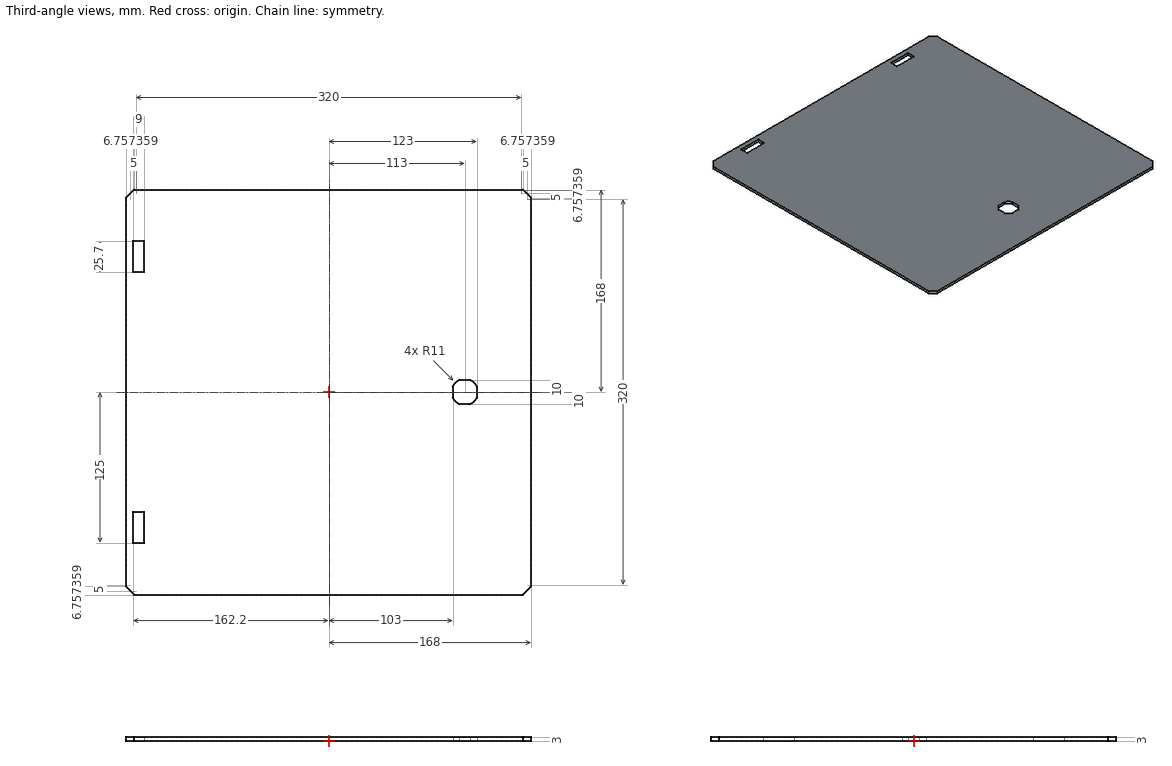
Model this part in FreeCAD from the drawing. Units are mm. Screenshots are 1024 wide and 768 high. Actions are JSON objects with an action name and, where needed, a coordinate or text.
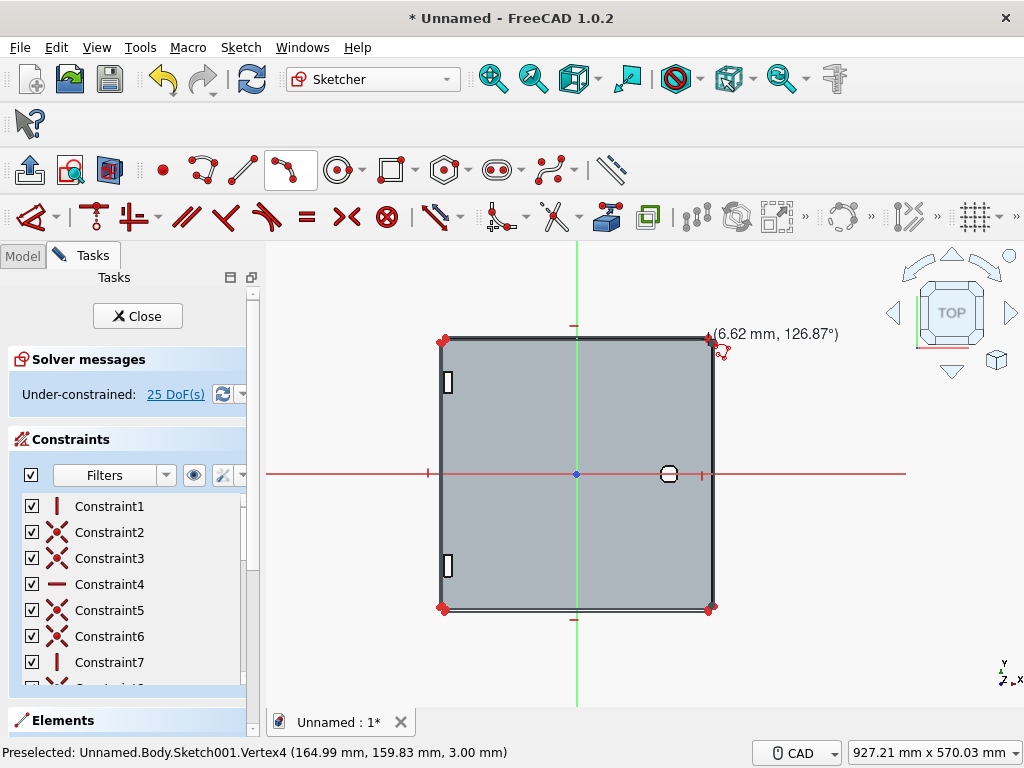
{"action": "scroll", "coordinate": [712, 605], "scroll_direction": "up", "scroll_amount": 10}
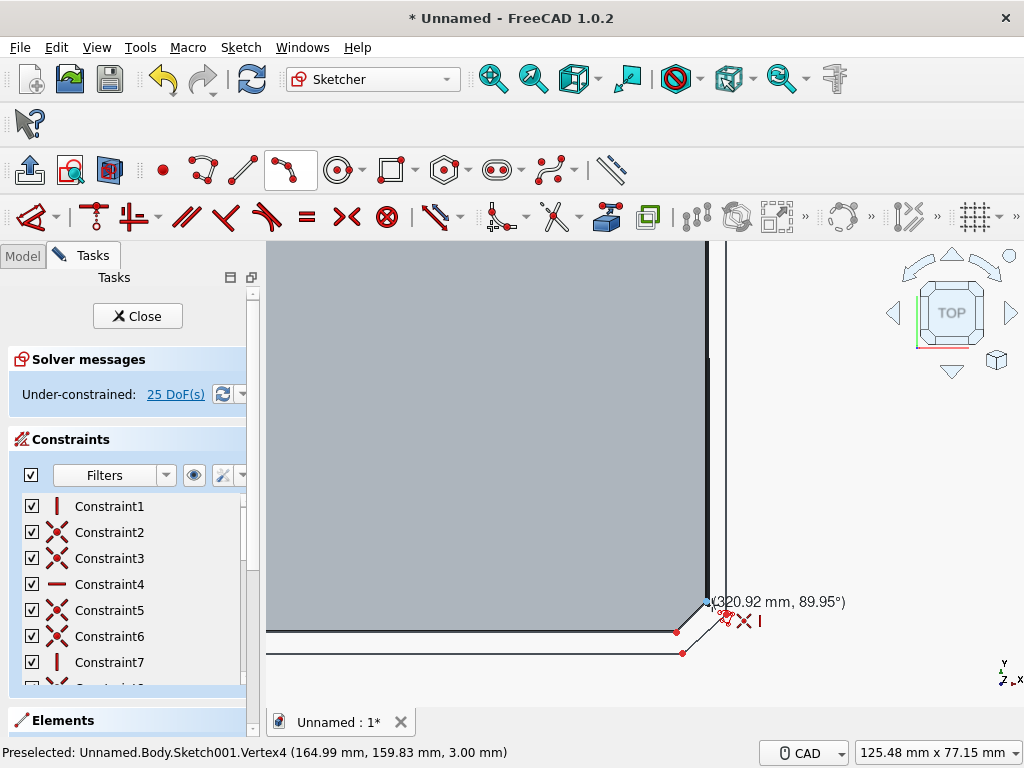
{"action": "left_click", "coordinate": [707, 601]}
{"action": "key", "text": "Escape"}
{"action": "key", "text": "Escape"}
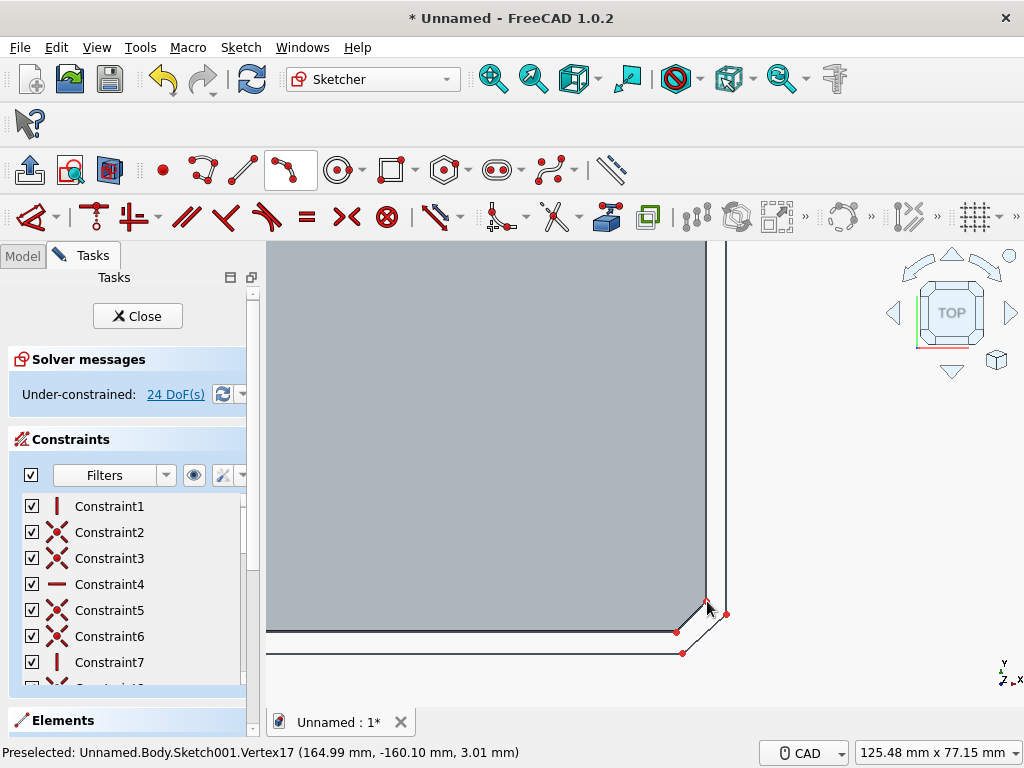
{"action": "scroll", "coordinate": [712, 605], "scroll_direction": "down", "scroll_amount": 10}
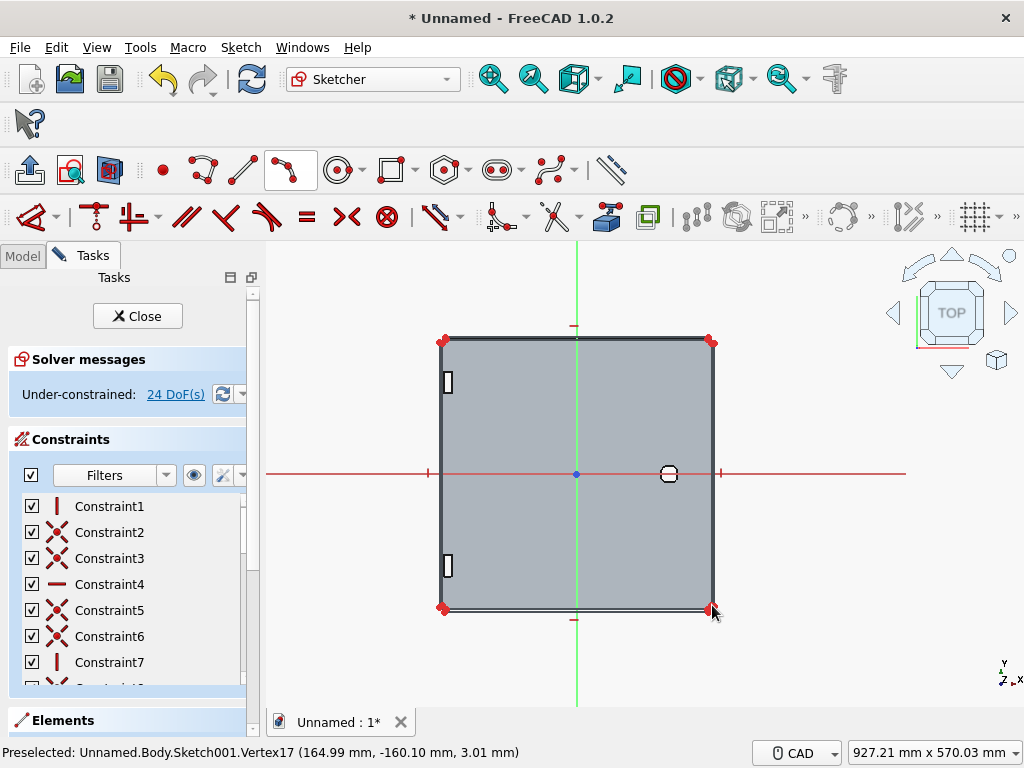
{"action": "scroll", "coordinate": [714, 343], "scroll_direction": "up", "scroll_amount": 8}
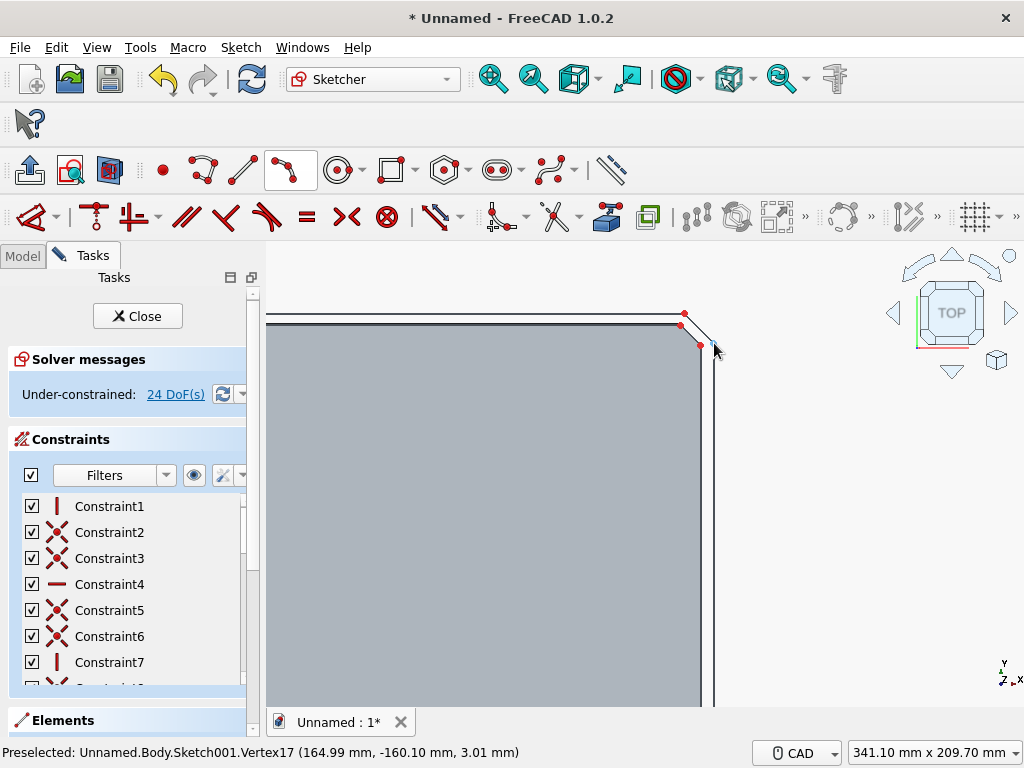
{"action": "left_click", "coordinate": [714, 344]}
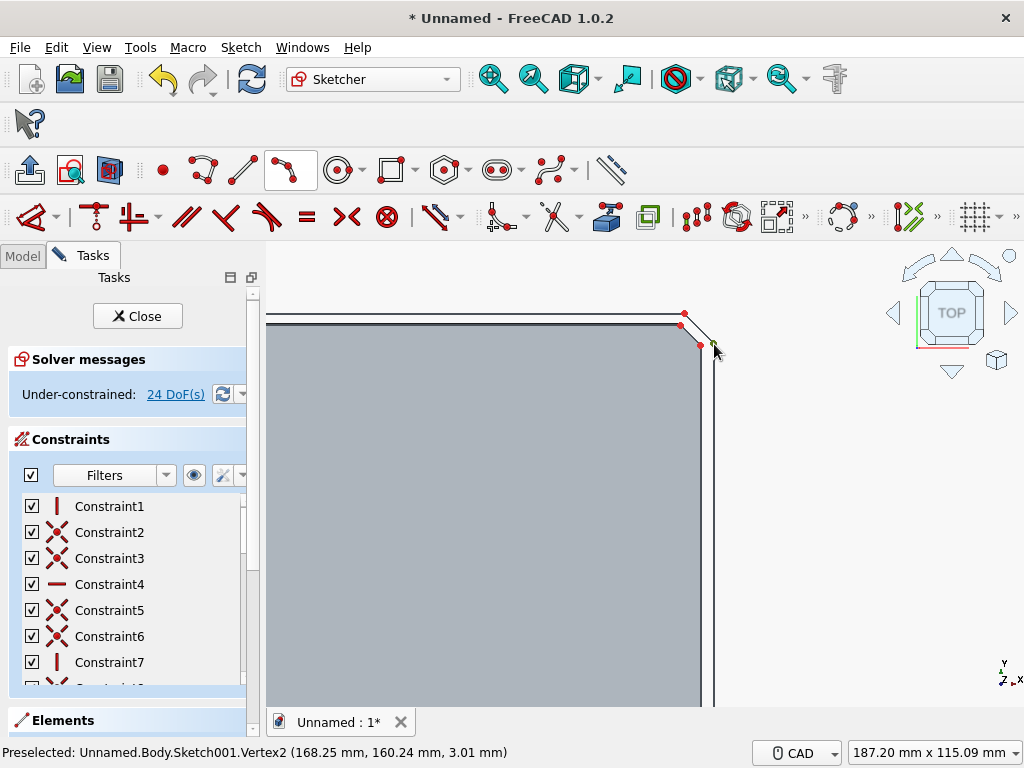
{"action": "scroll", "coordinate": [714, 343], "scroll_direction": "down", "scroll_amount": 8}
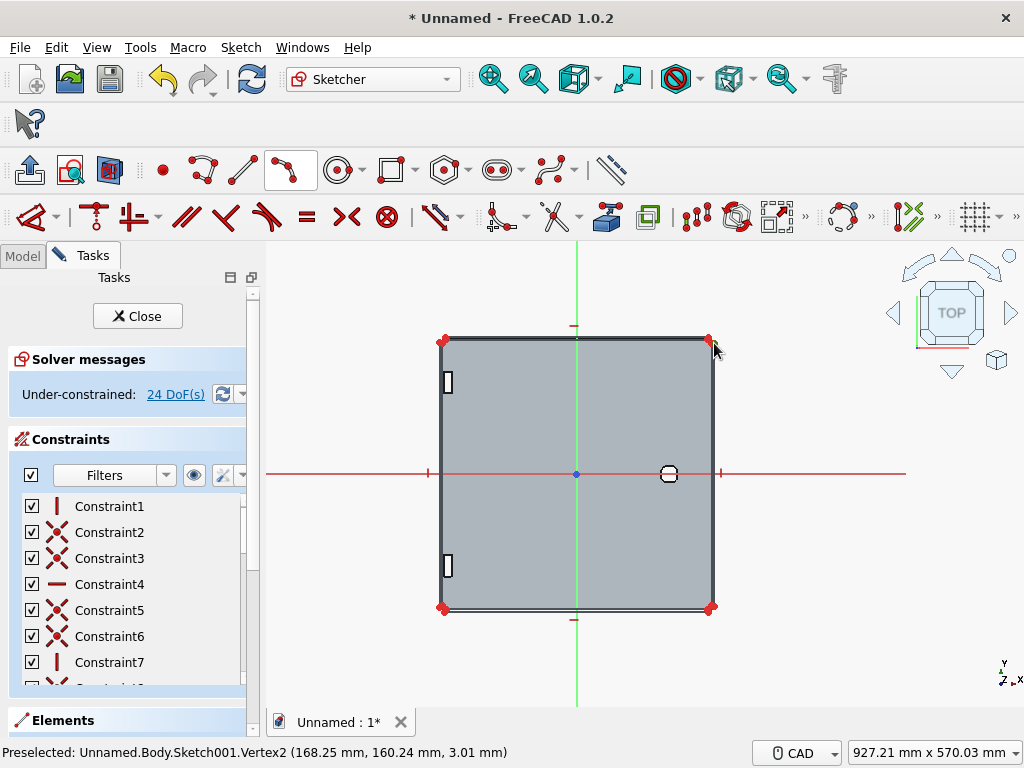
{"action": "scroll", "coordinate": [440, 343], "scroll_direction": "up", "scroll_amount": 9}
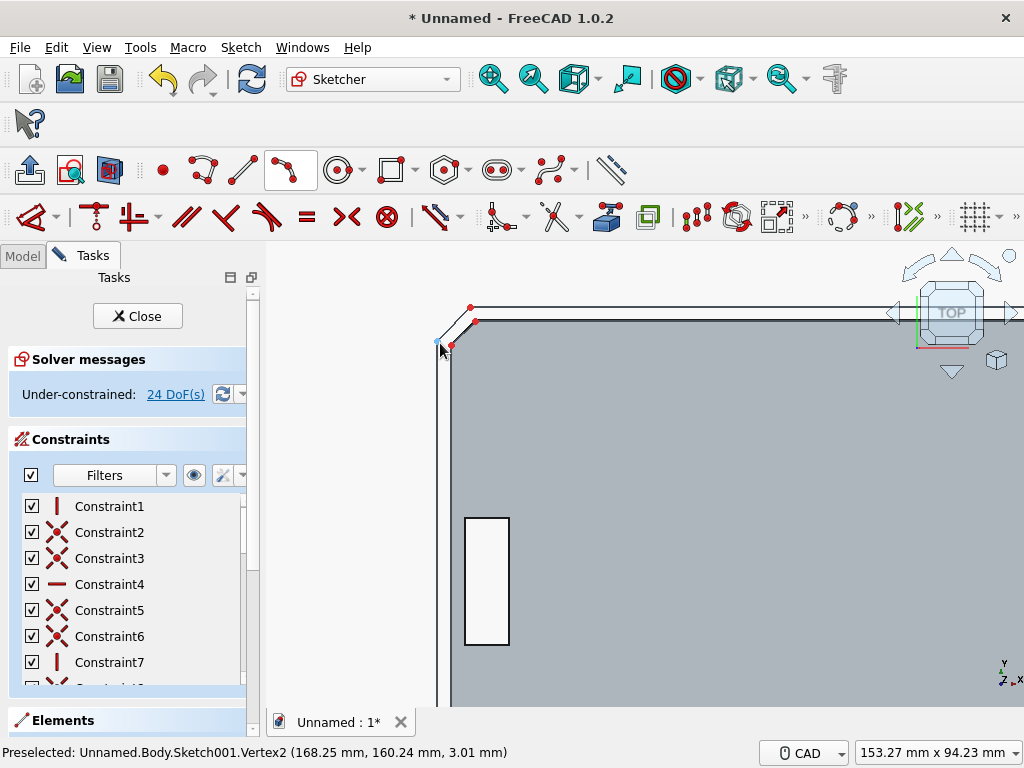
{"action": "left_click", "coordinate": [437, 342]}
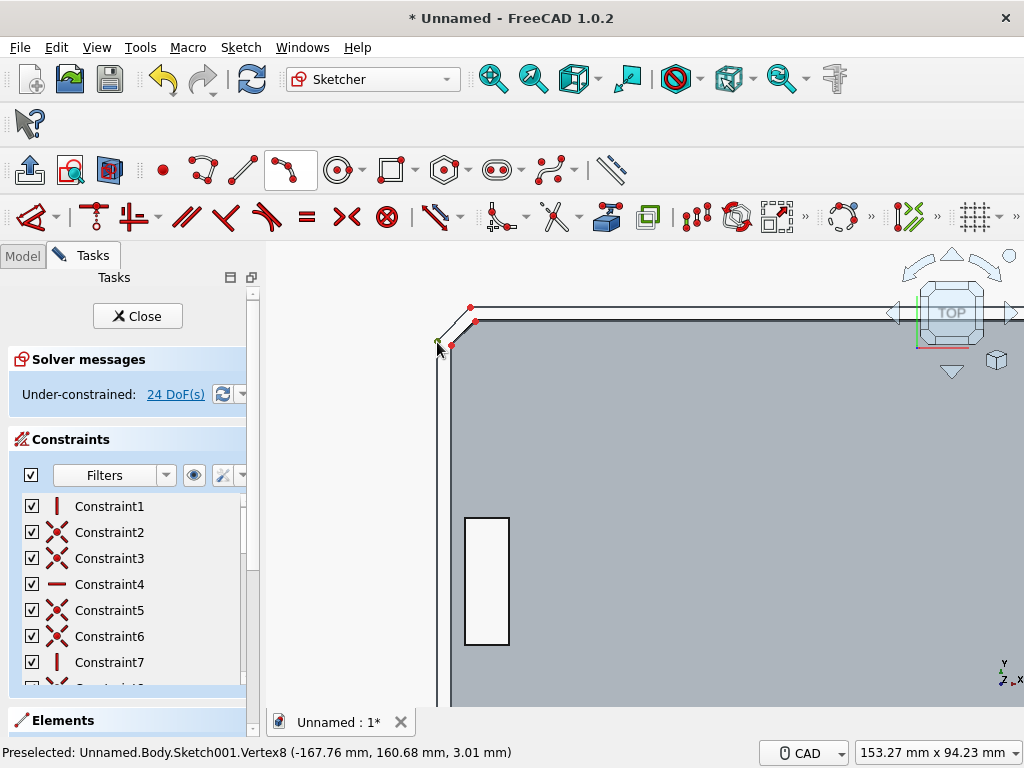
{"action": "scroll", "coordinate": [440, 343], "scroll_direction": "down", "scroll_amount": 9}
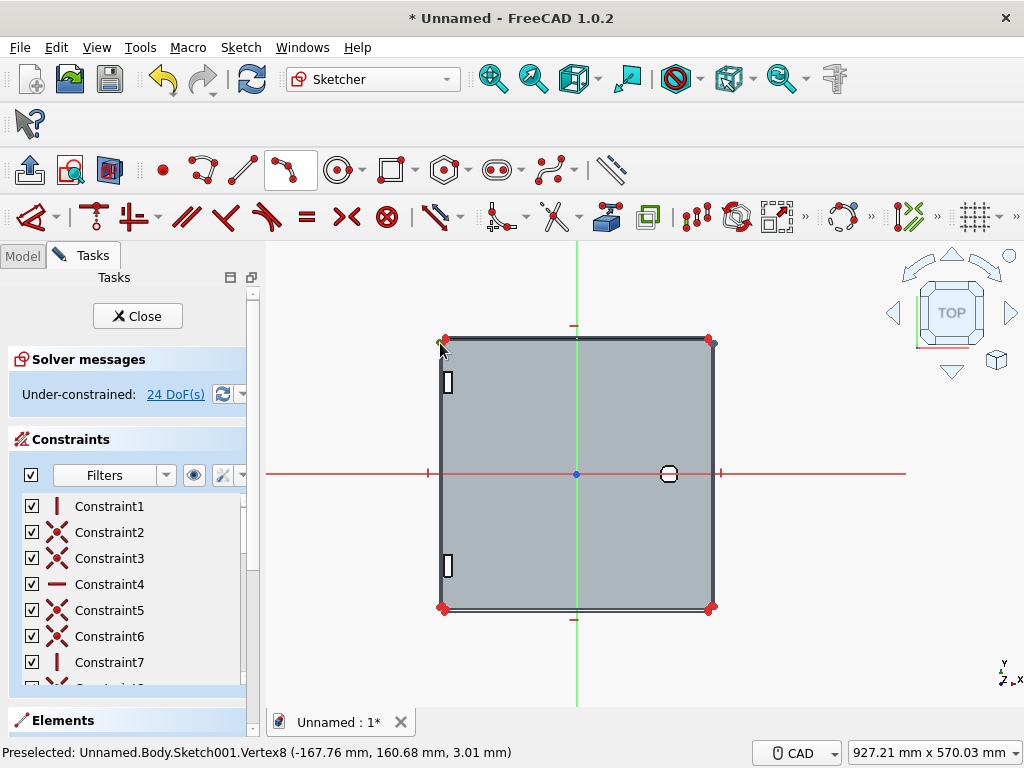
{"action": "left_click", "coordinate": [577, 650]}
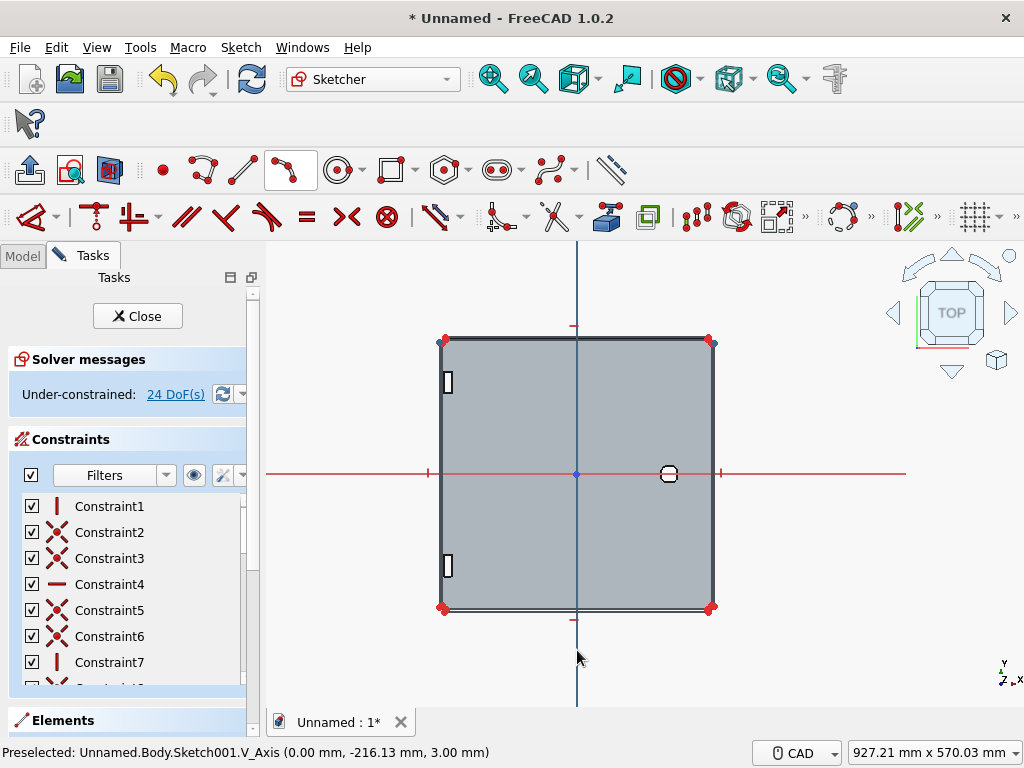
{"action": "left_click", "coordinate": [348, 218]}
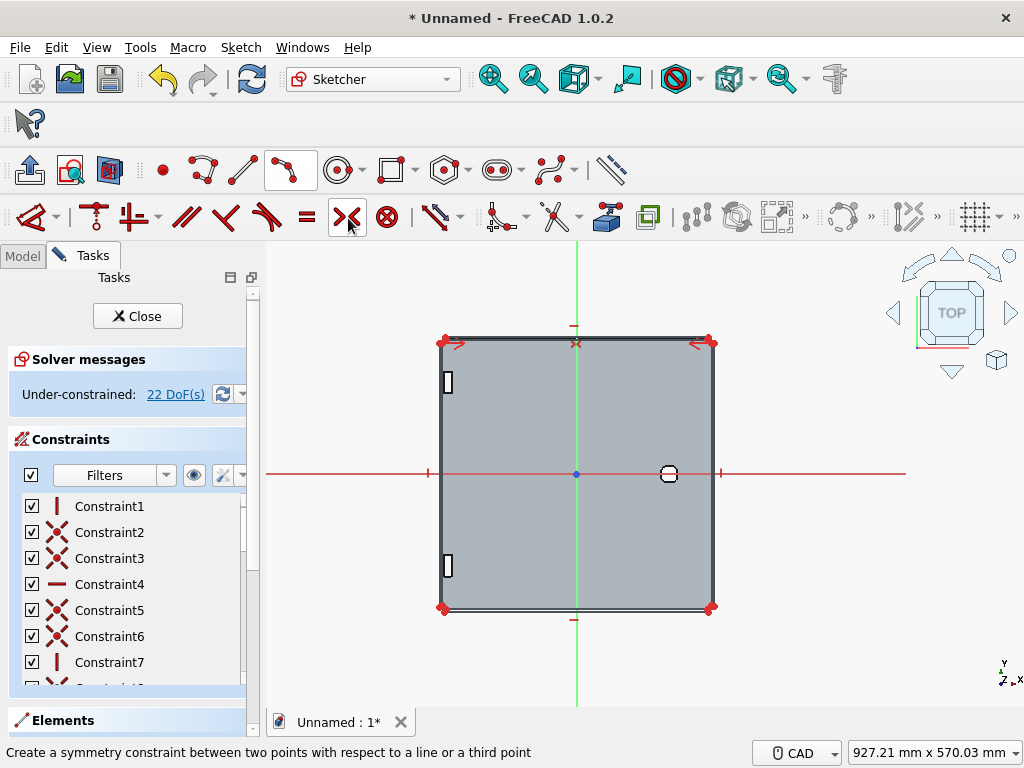
{"action": "scroll", "coordinate": [445, 337], "scroll_direction": "up", "scroll_amount": 8}